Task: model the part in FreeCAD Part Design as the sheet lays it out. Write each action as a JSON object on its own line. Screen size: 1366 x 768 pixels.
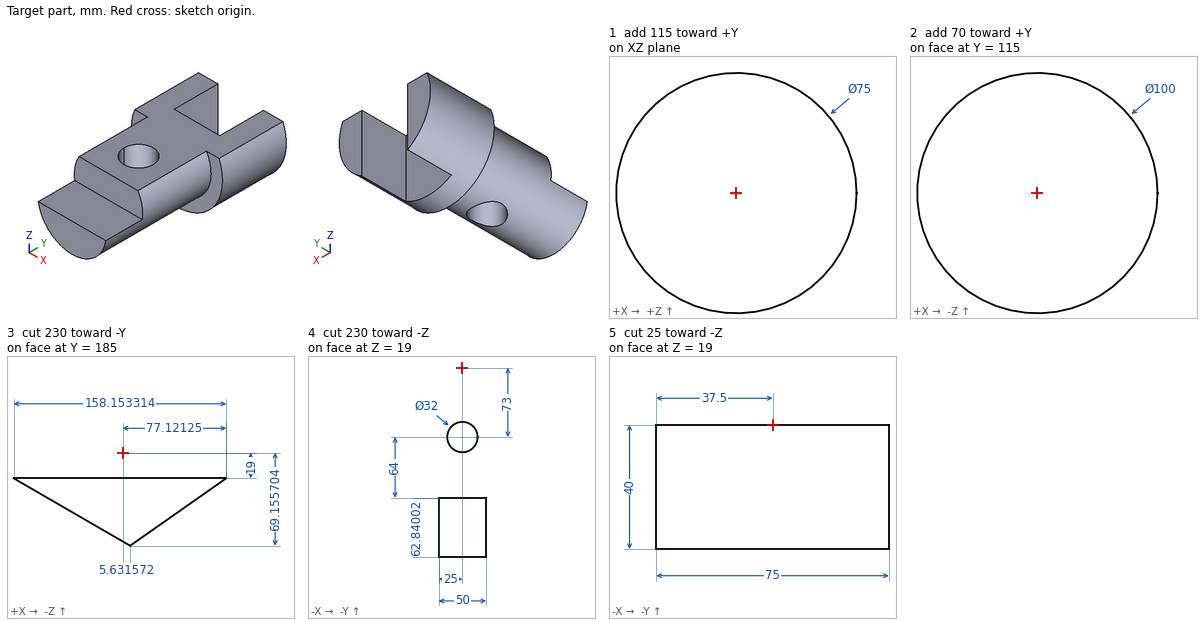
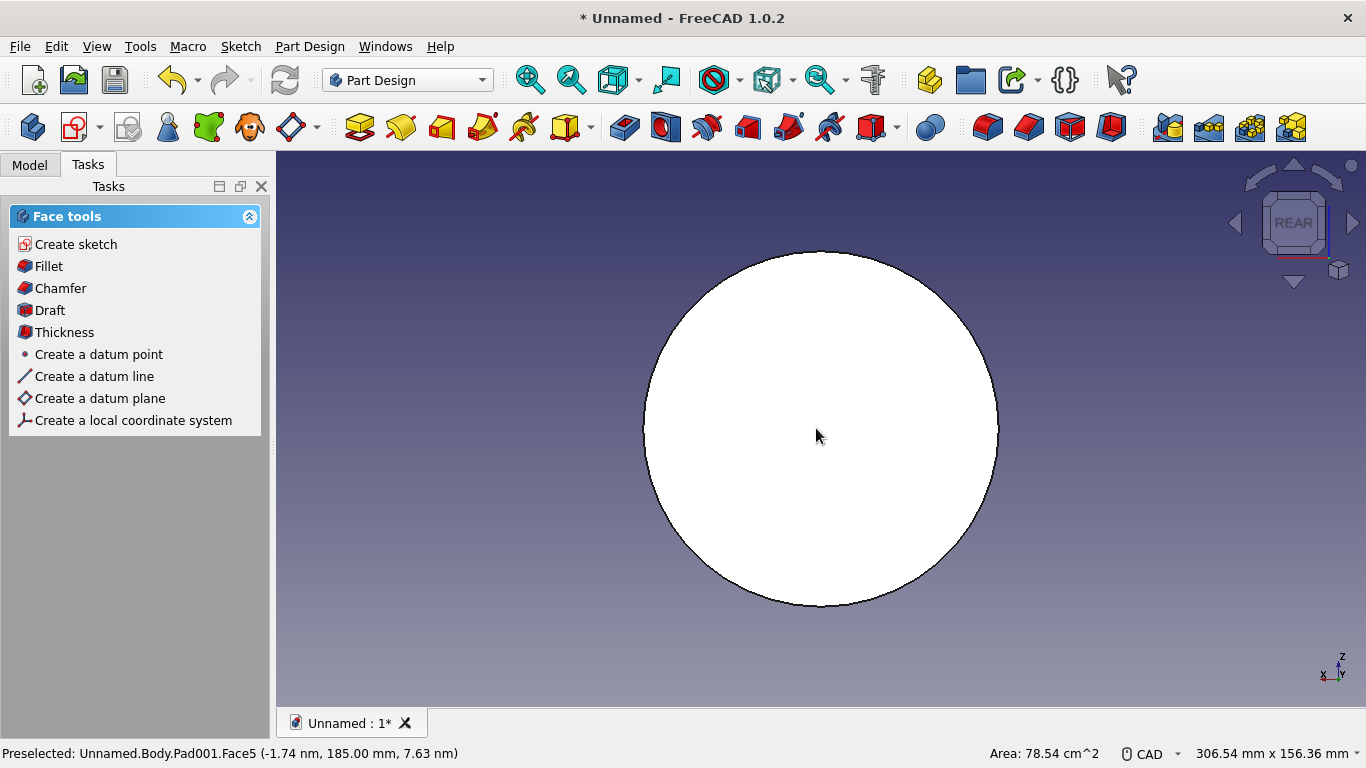
{"action": "left_click", "coordinate": [74, 128]}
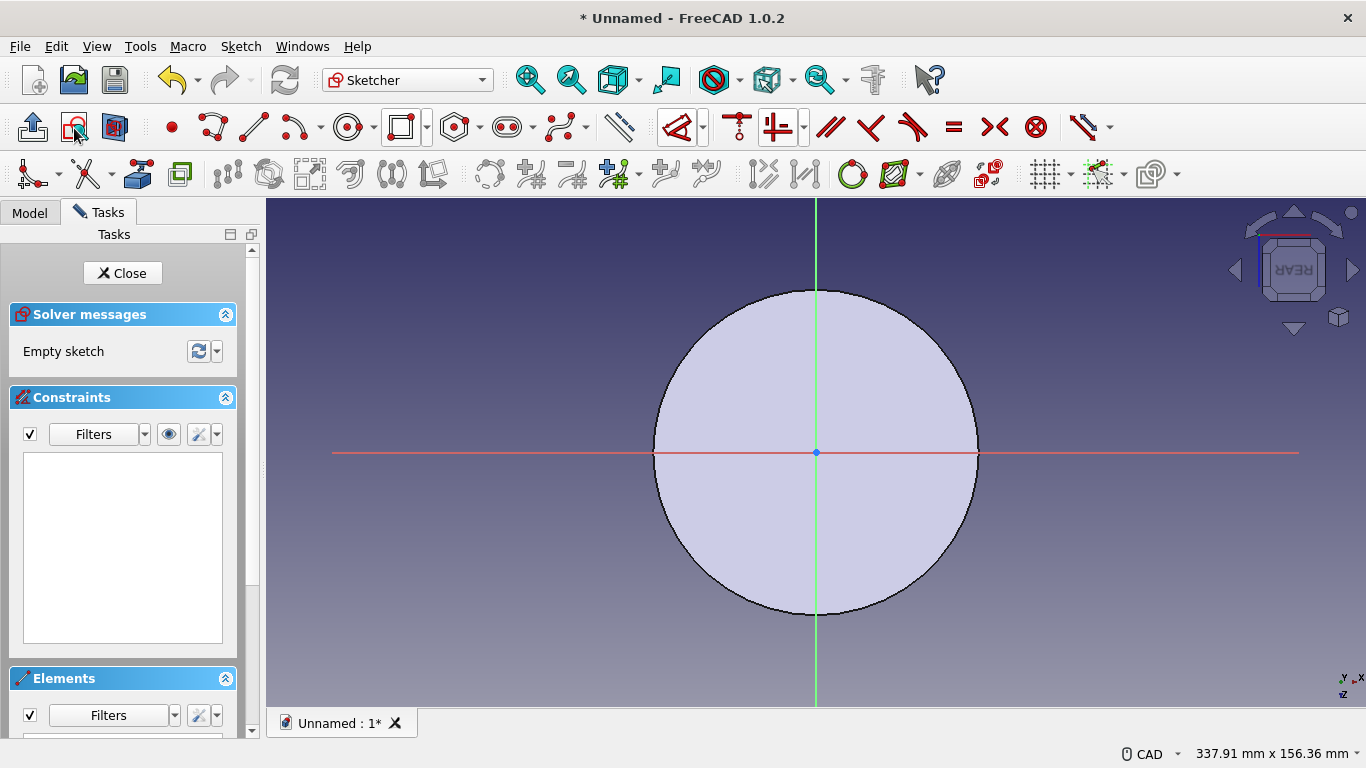
{"action": "scroll", "coordinate": [467, 226], "scroll_direction": "down", "scroll_amount": 1}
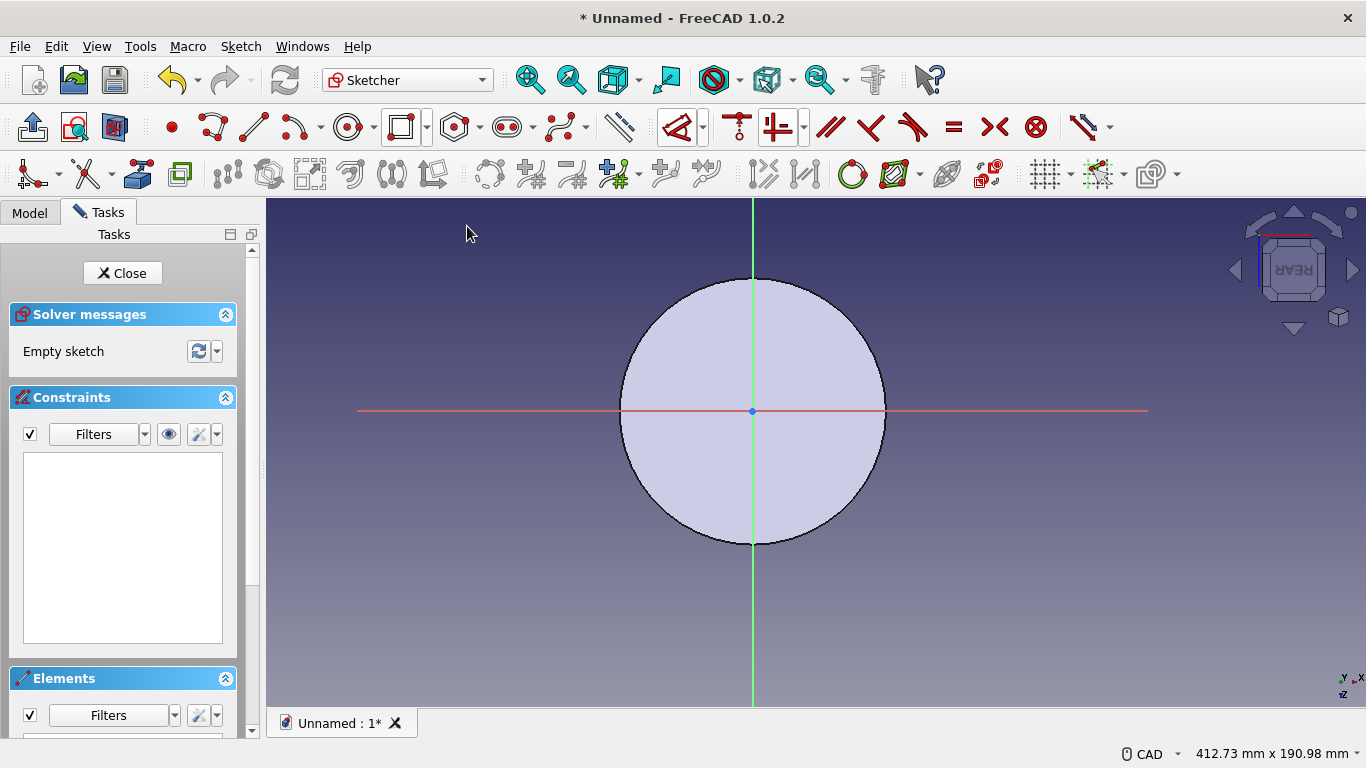
{"action": "scroll", "coordinate": [748, 608], "scroll_direction": "up", "scroll_amount": 2}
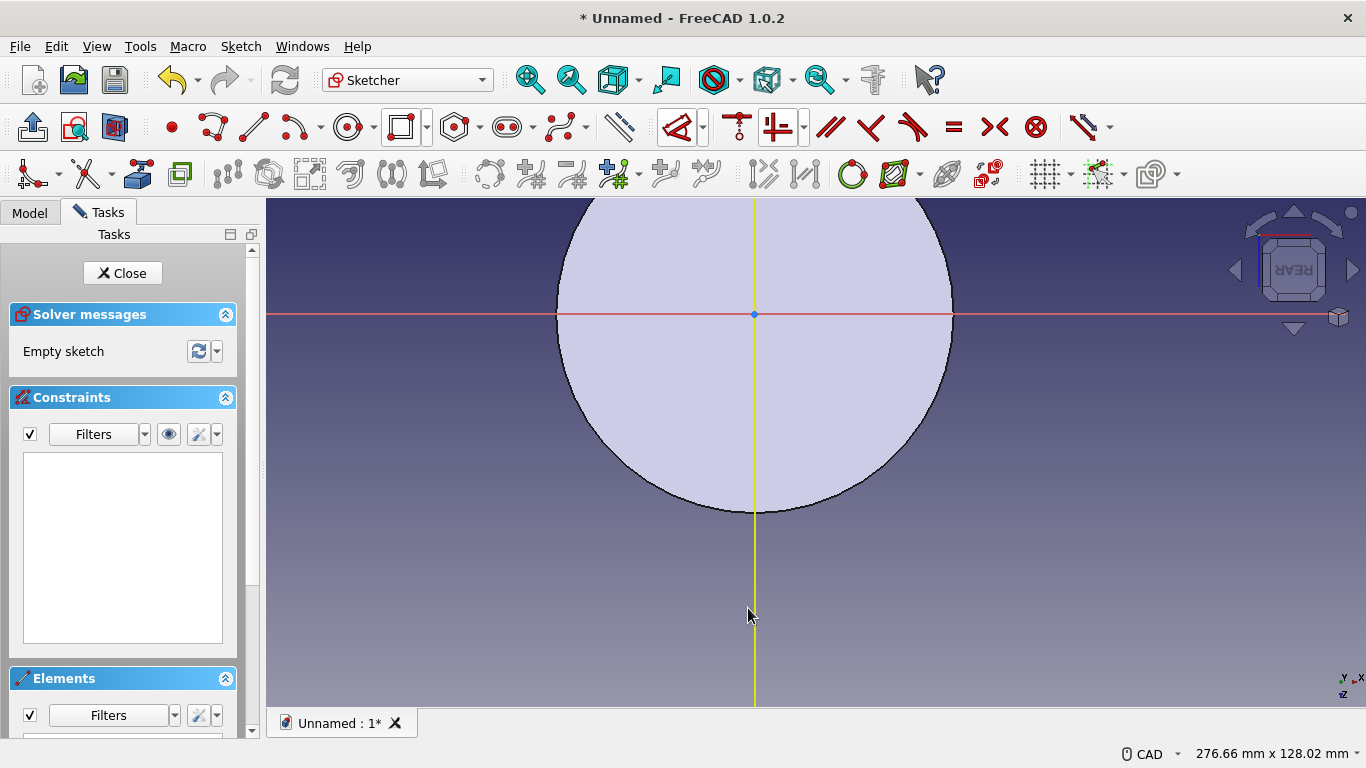
{"action": "left_click", "coordinate": [213, 128]}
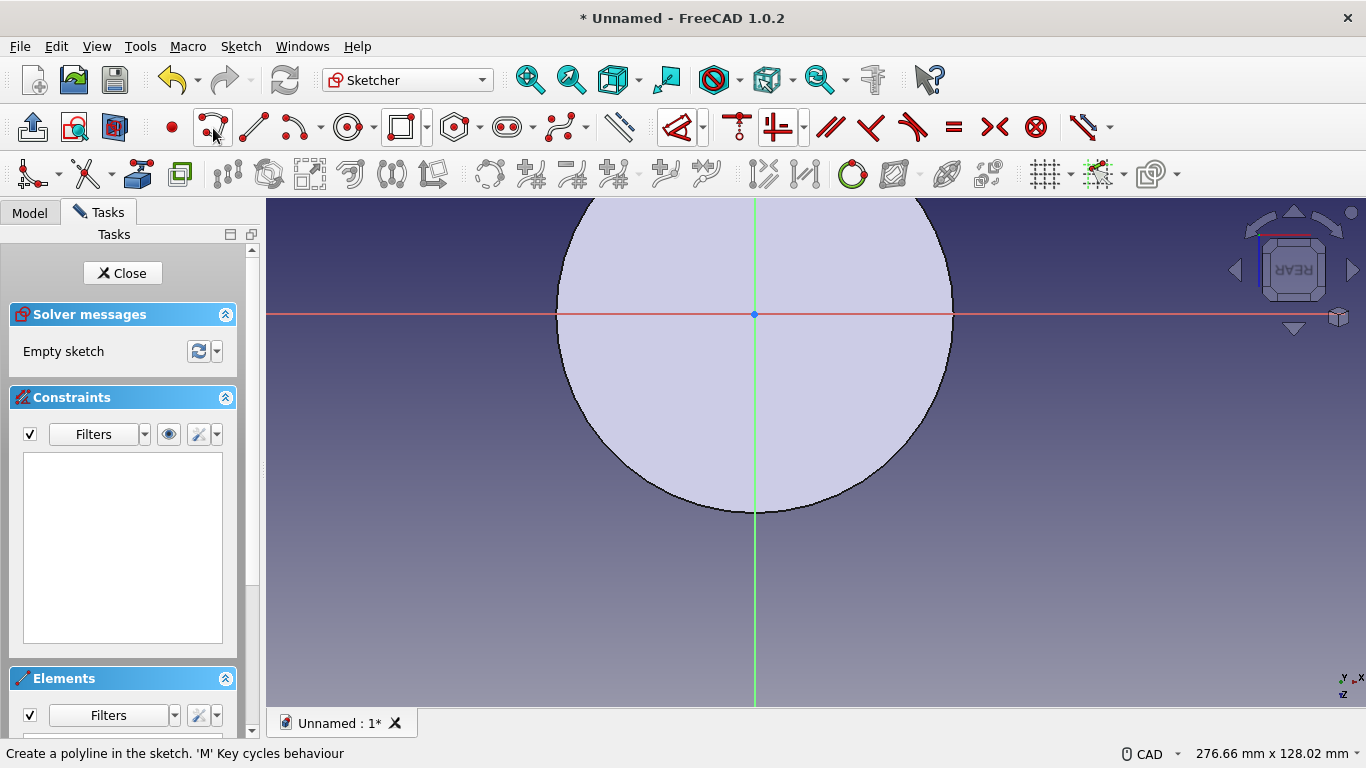
{"action": "left_click", "coordinate": [777, 589]}
{"action": "left_click", "coordinate": [1062, 390]}
{"action": "left_click", "coordinate": [433, 390]}
{"action": "left_click", "coordinate": [777, 590]}
{"action": "key", "text": "Escape"}
{"action": "key", "text": "Escape"}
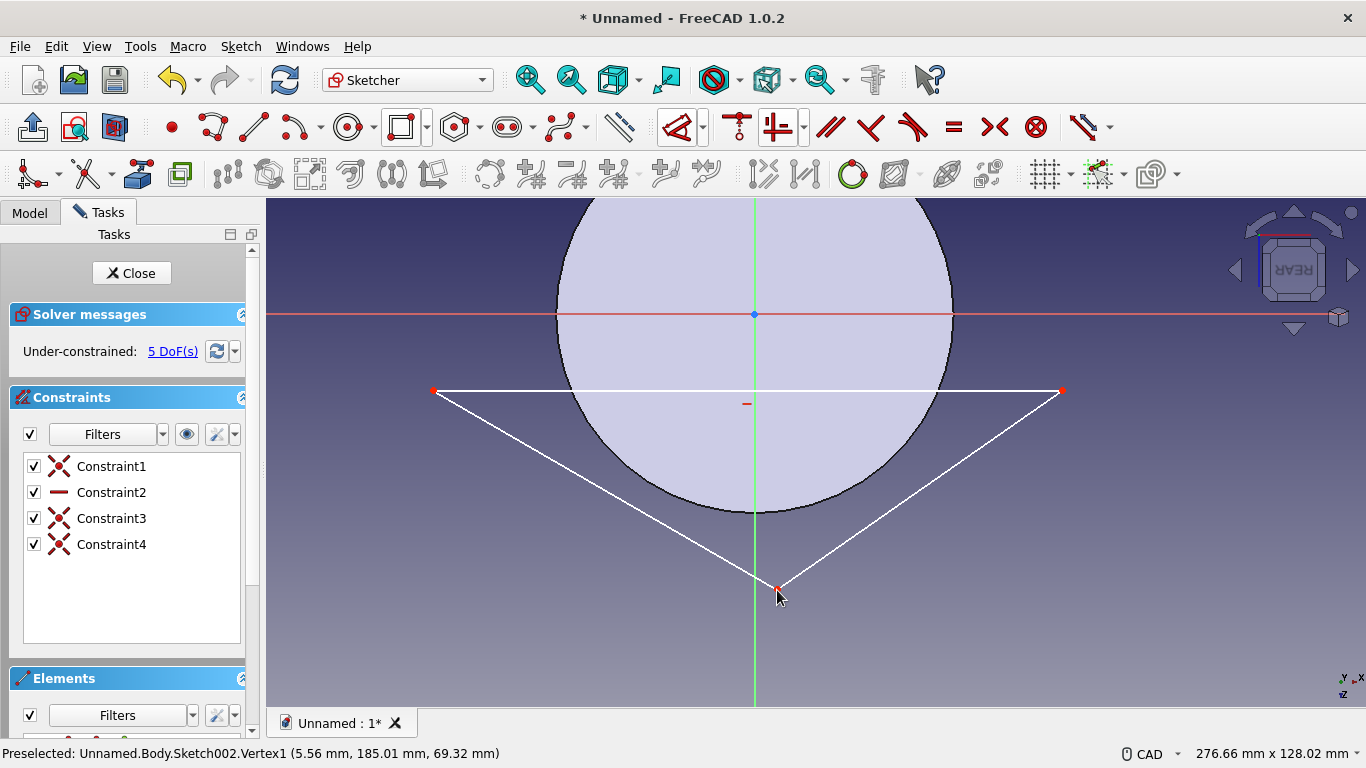
{"action": "left_click", "coordinate": [1062, 391]}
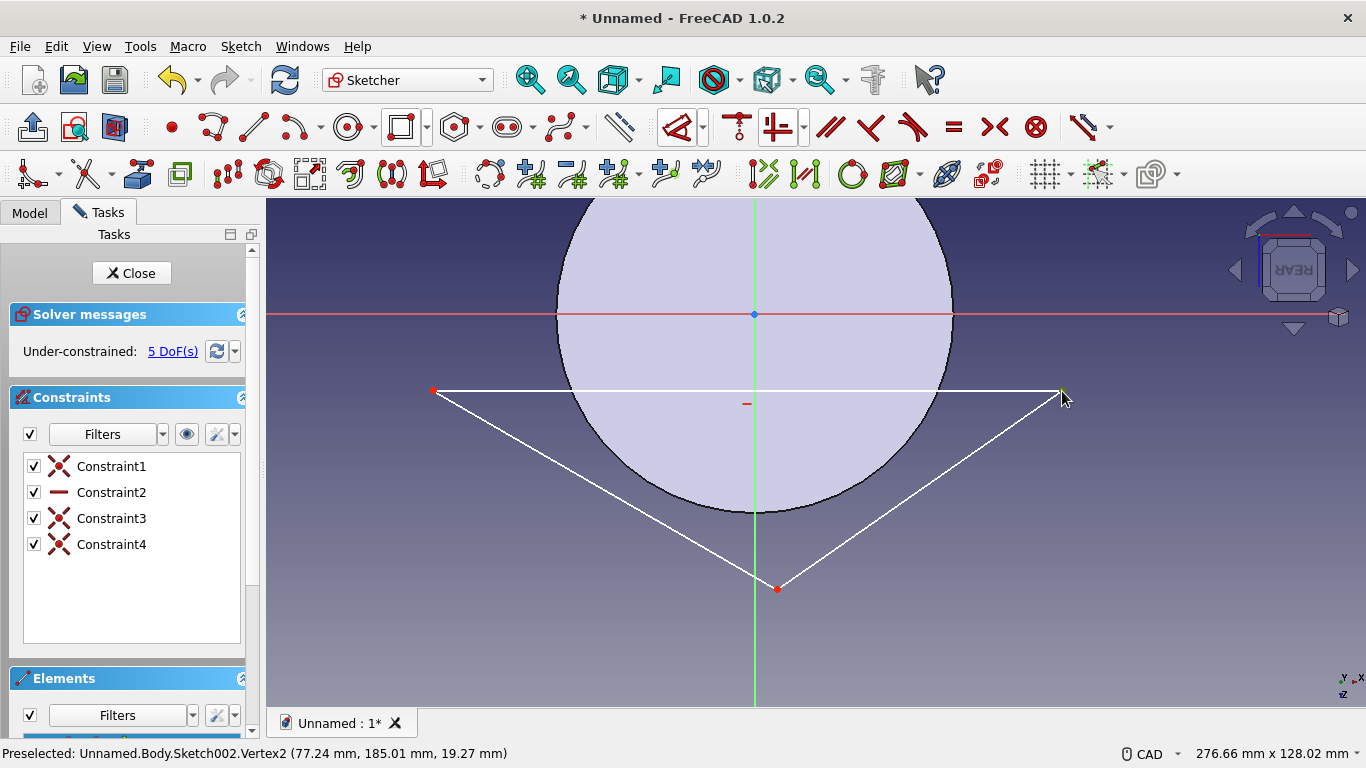
{"action": "key", "text": "i"}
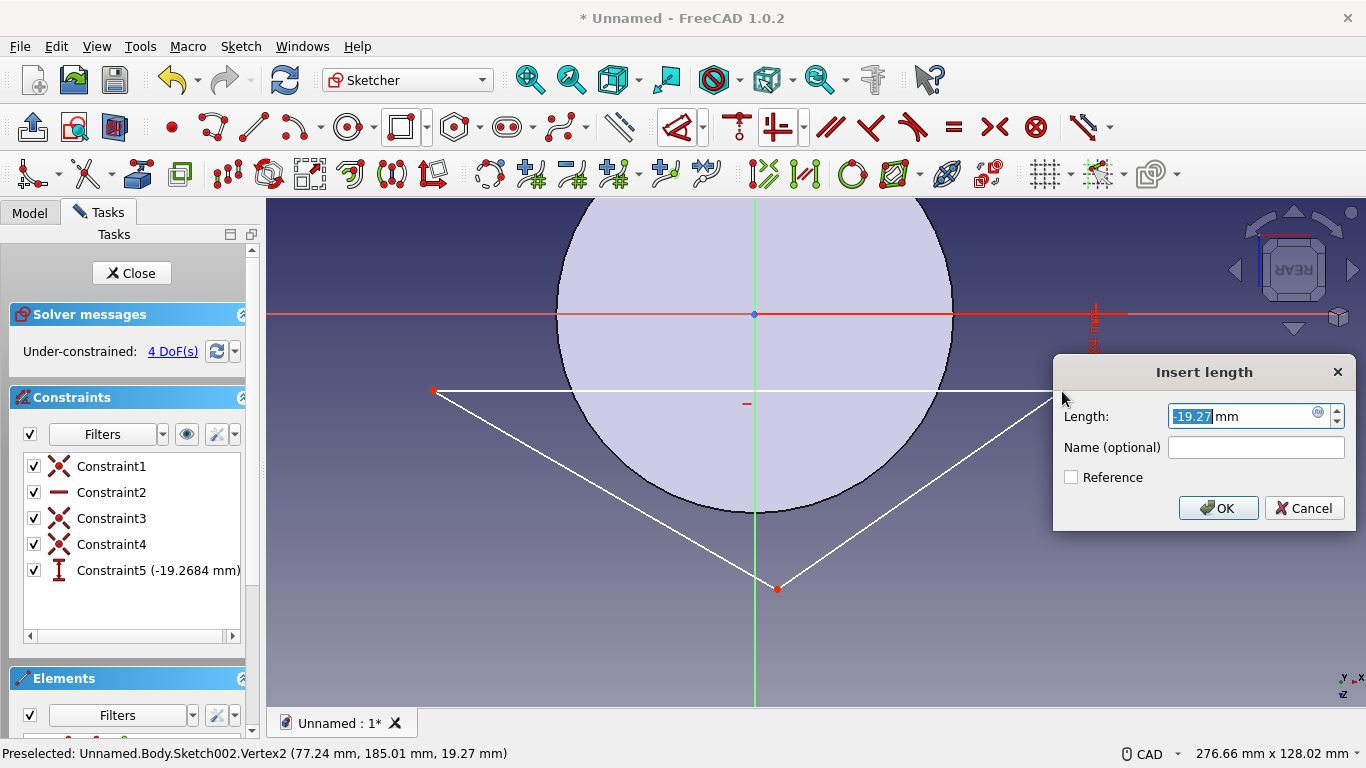
{"action": "type", "text": "-19"}
{"action": "key", "text": "Return"}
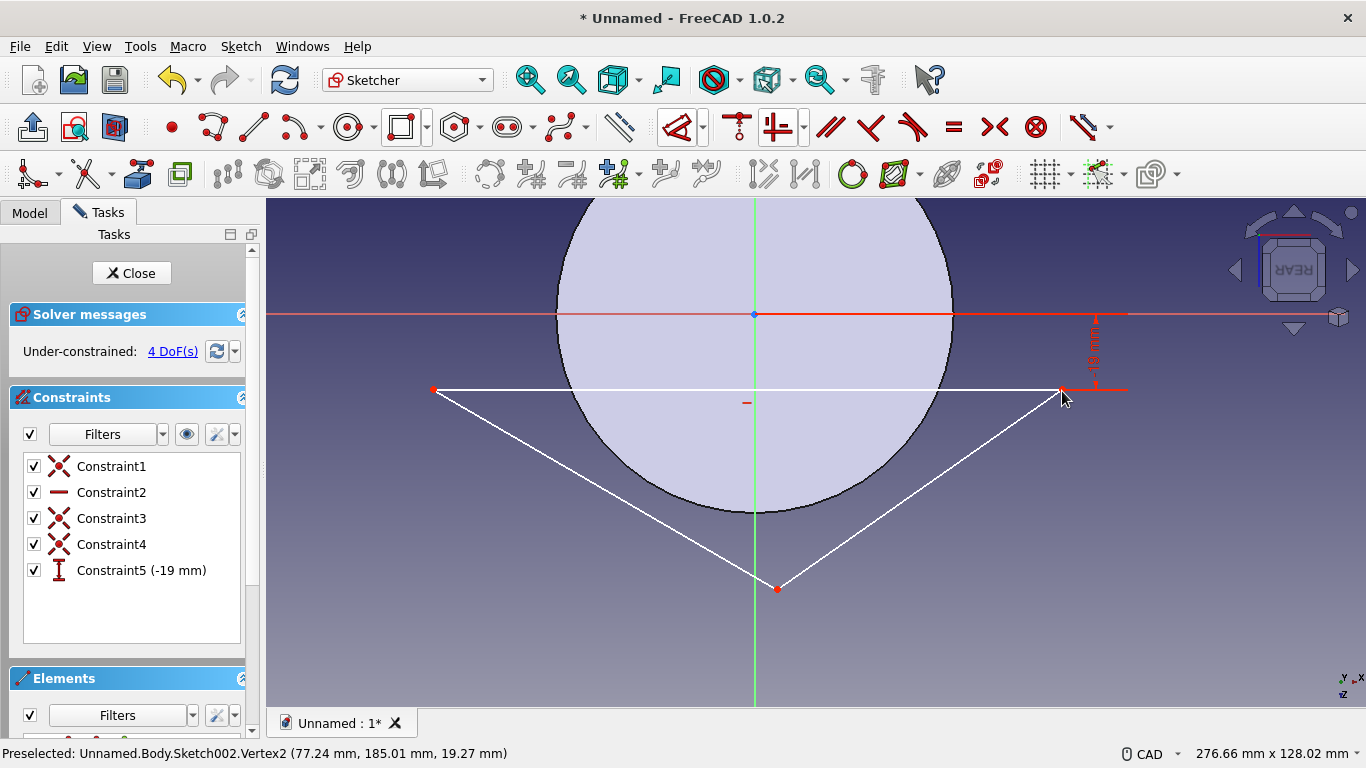
{"action": "scroll", "coordinate": [777, 590], "scroll_direction": "up", "scroll_amount": 3}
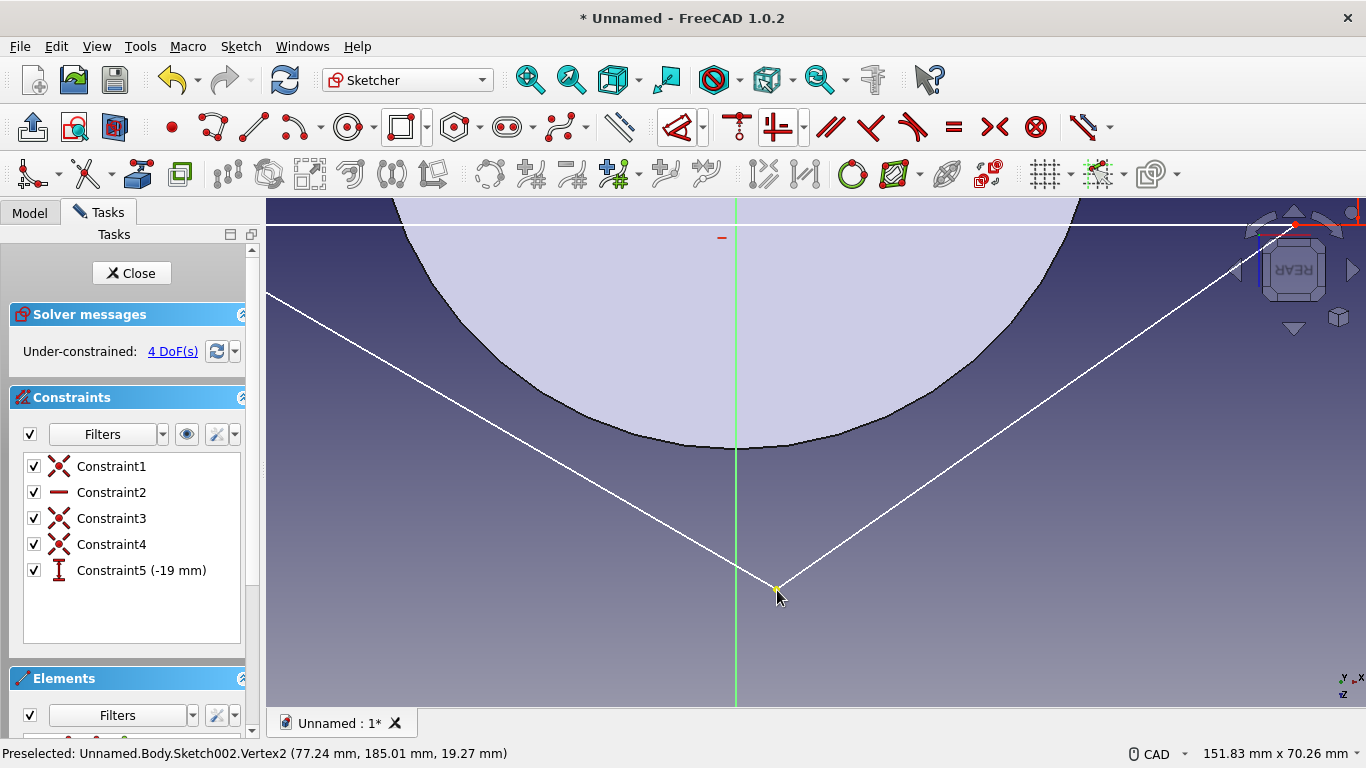
{"action": "left_click", "coordinate": [777, 589]}